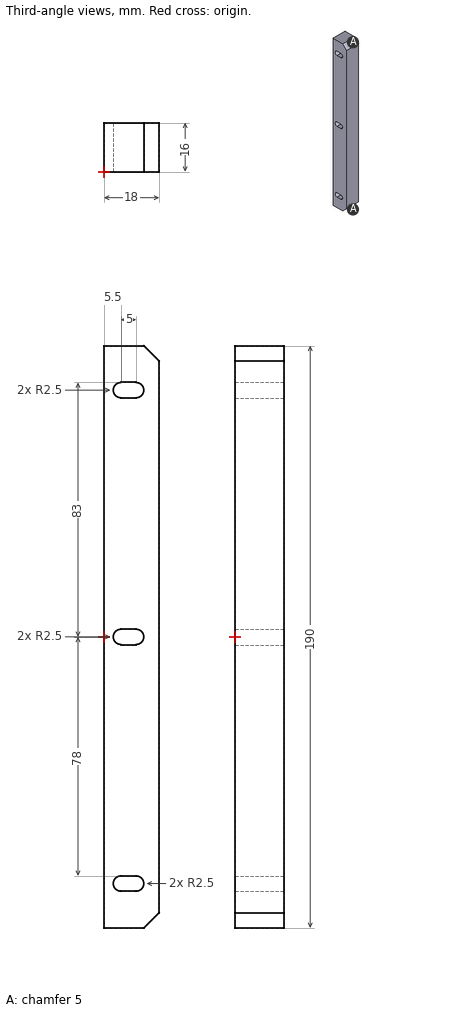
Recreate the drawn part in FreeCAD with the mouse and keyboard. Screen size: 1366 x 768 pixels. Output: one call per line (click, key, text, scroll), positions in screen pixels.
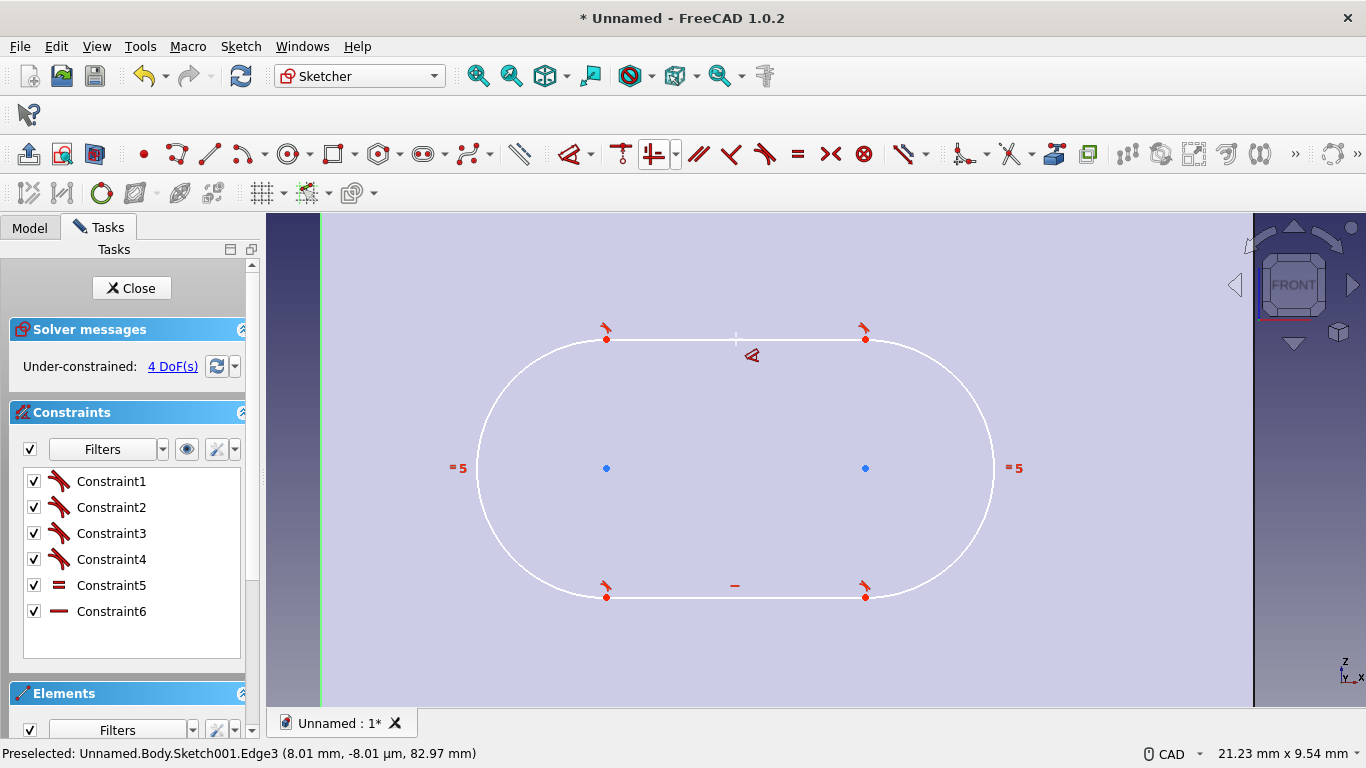
click(502, 393)
click(476, 374)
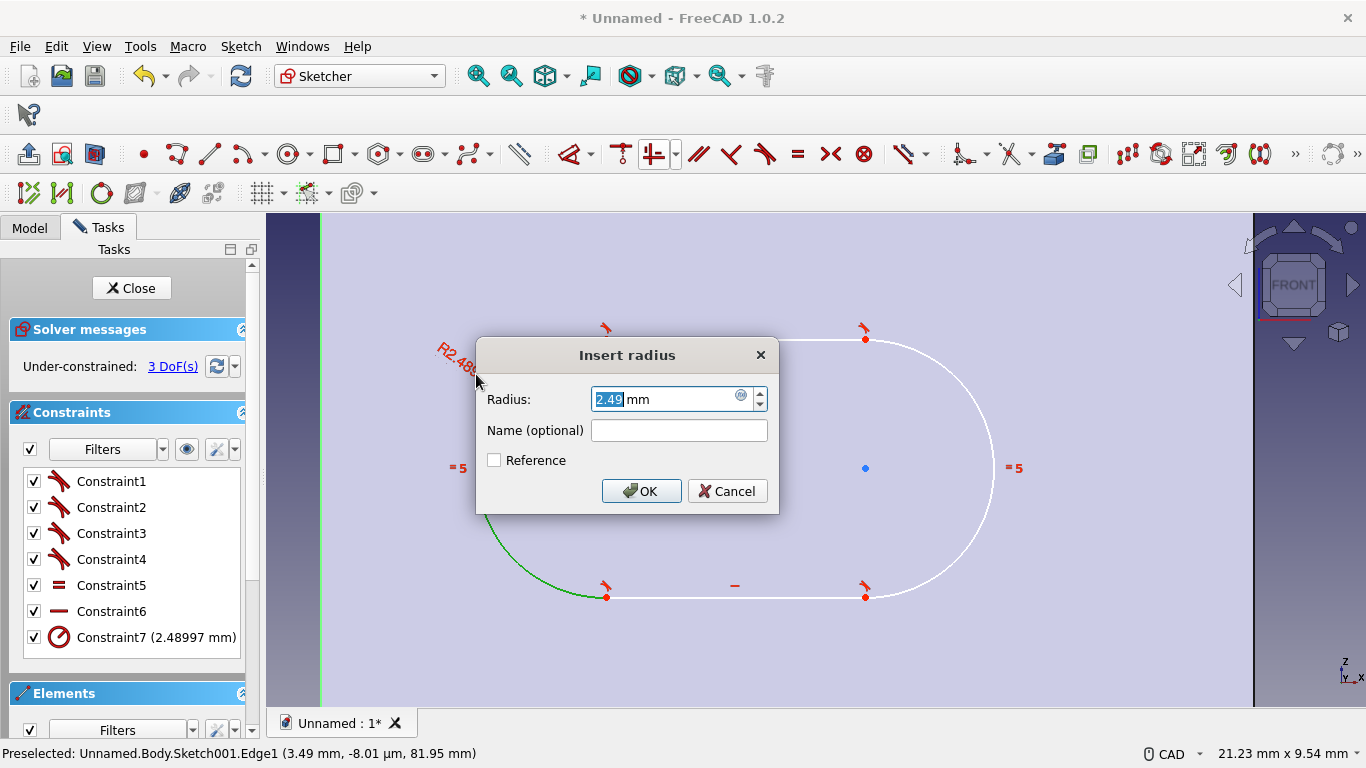
text(2.5)
key(Return)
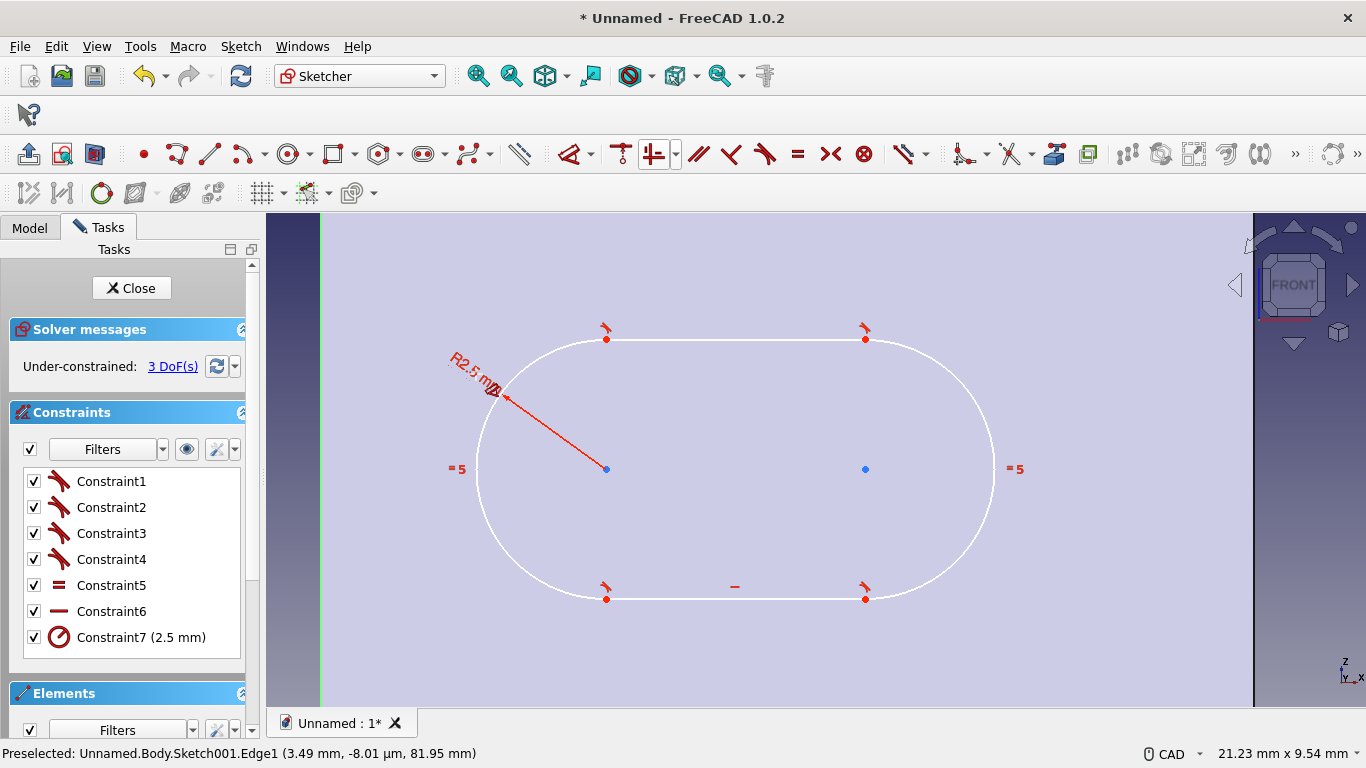
click(684, 340)
click(736, 306)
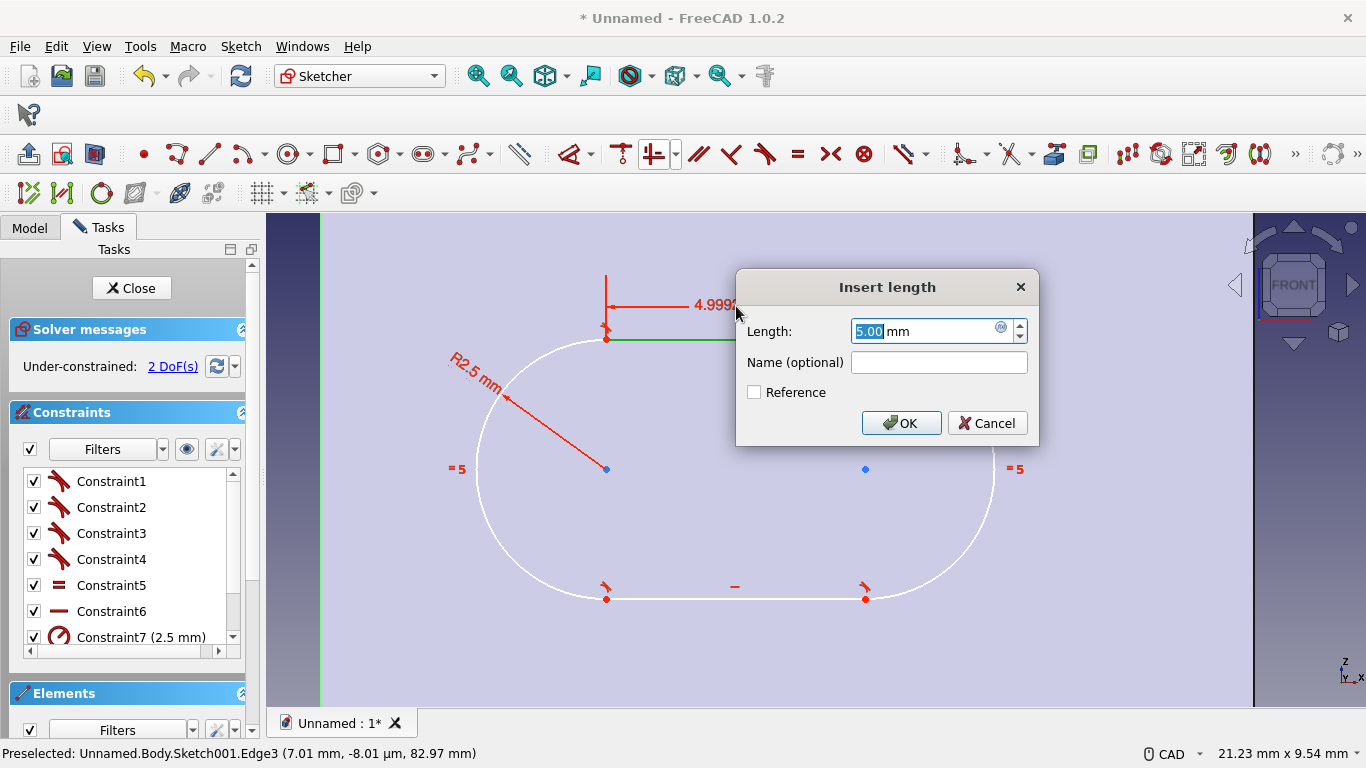
text(5)
key(Return)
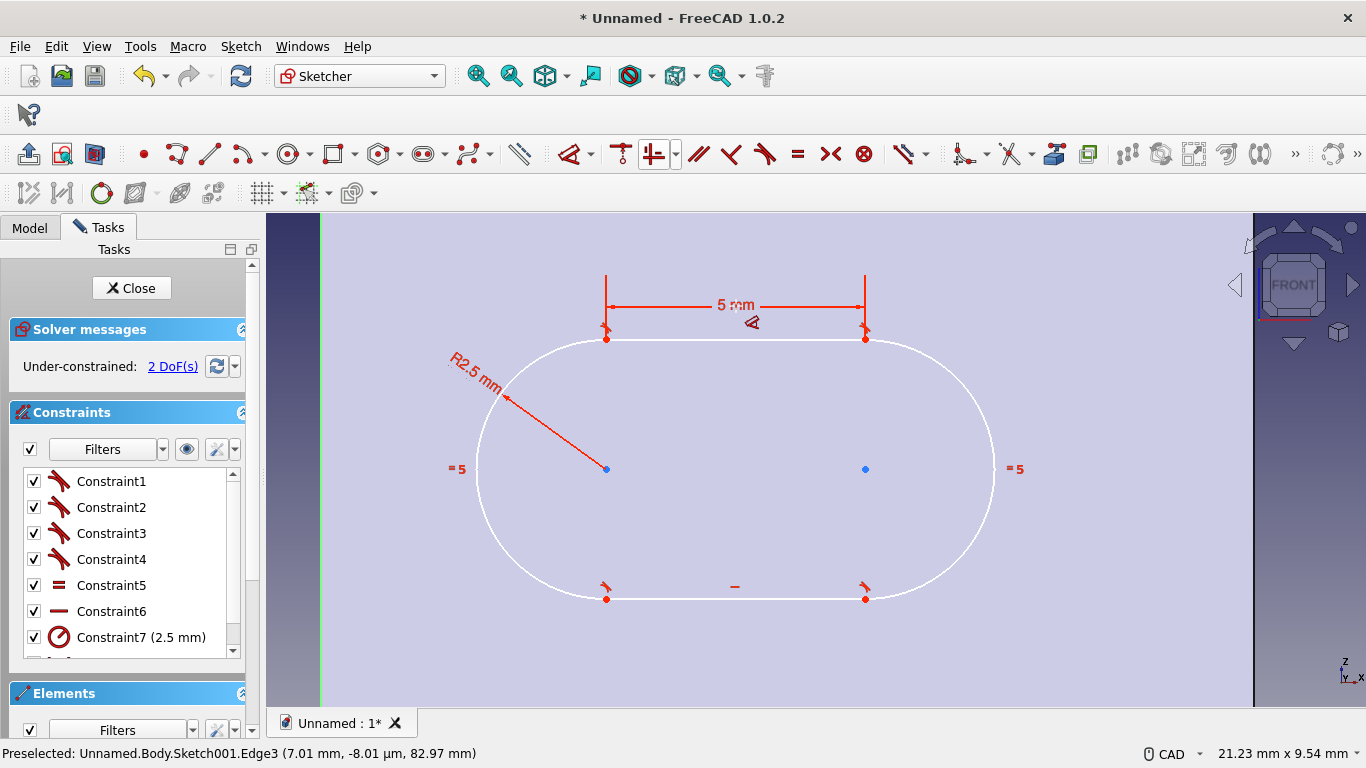
click(606, 340)
click(640, 509)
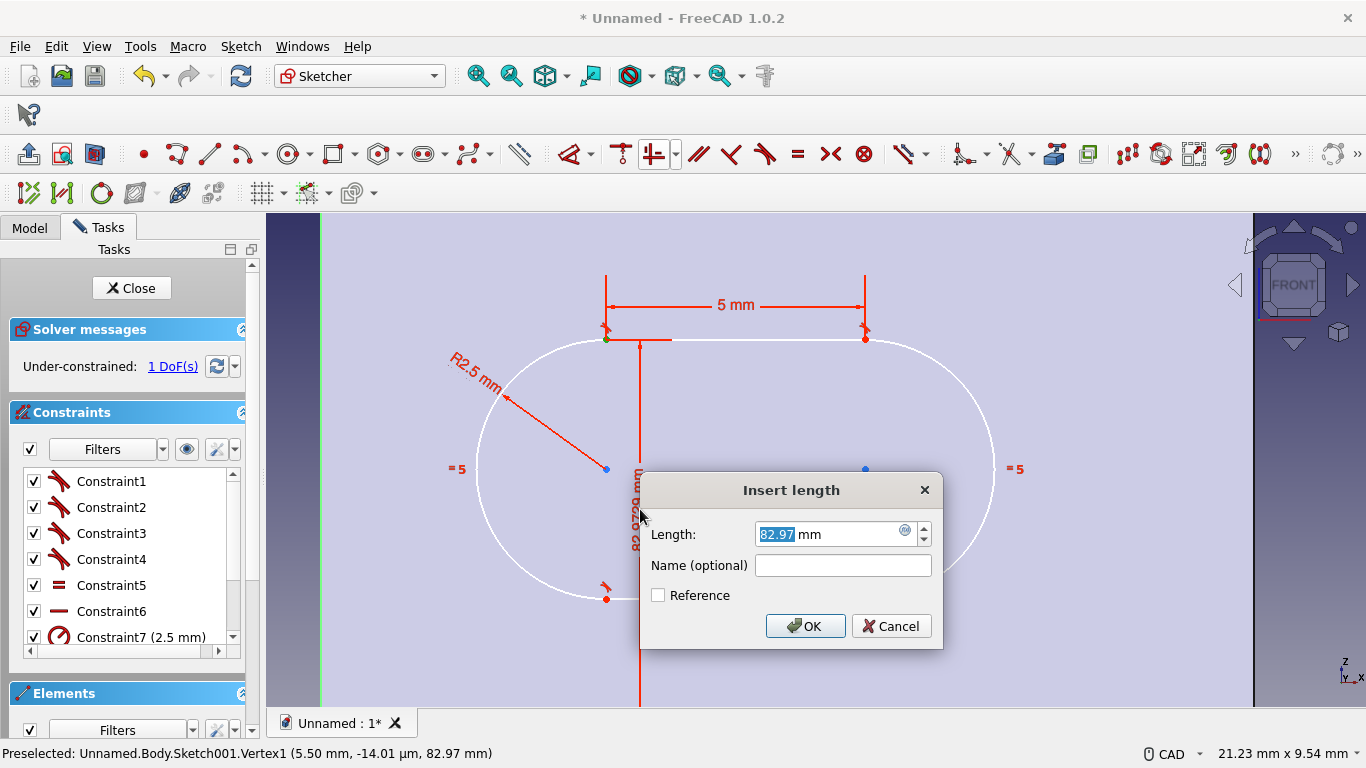
text(83)
key(Return)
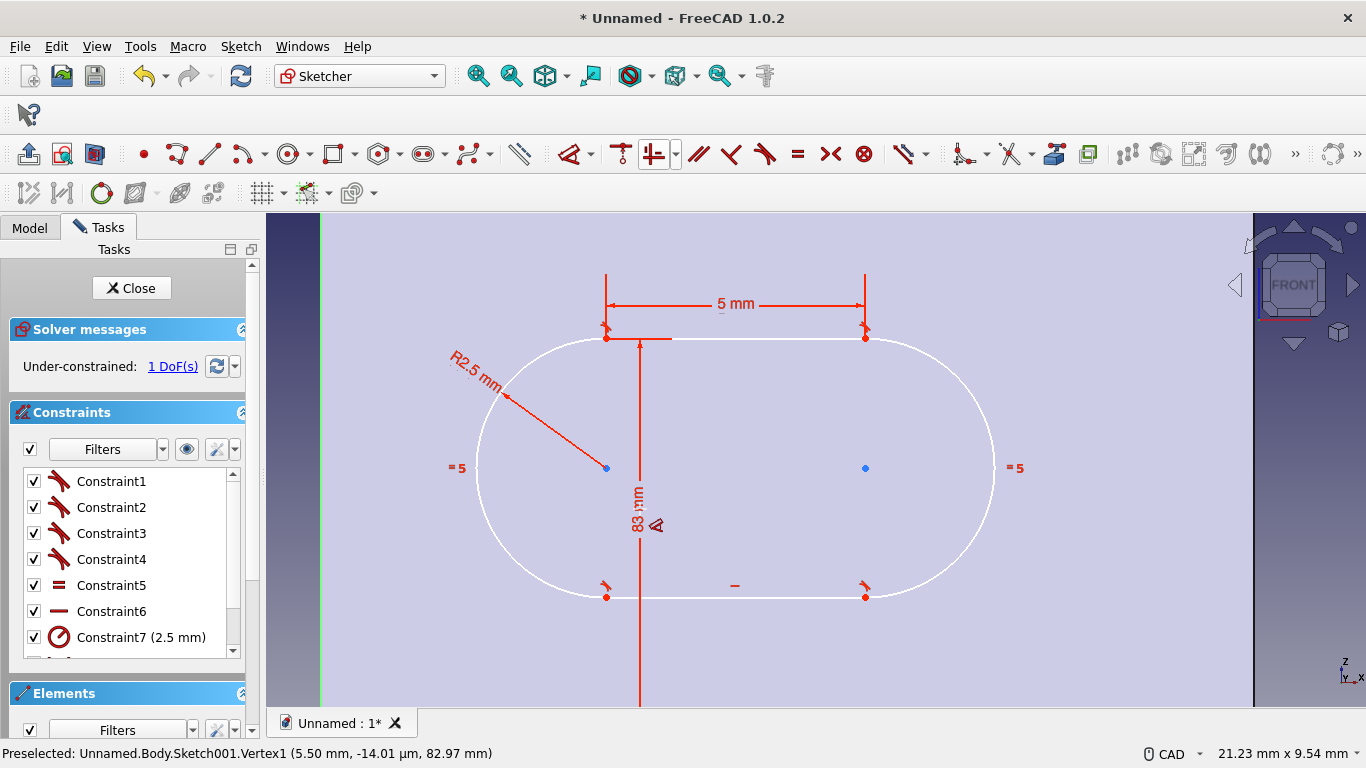
click(606, 339)
click(464, 305)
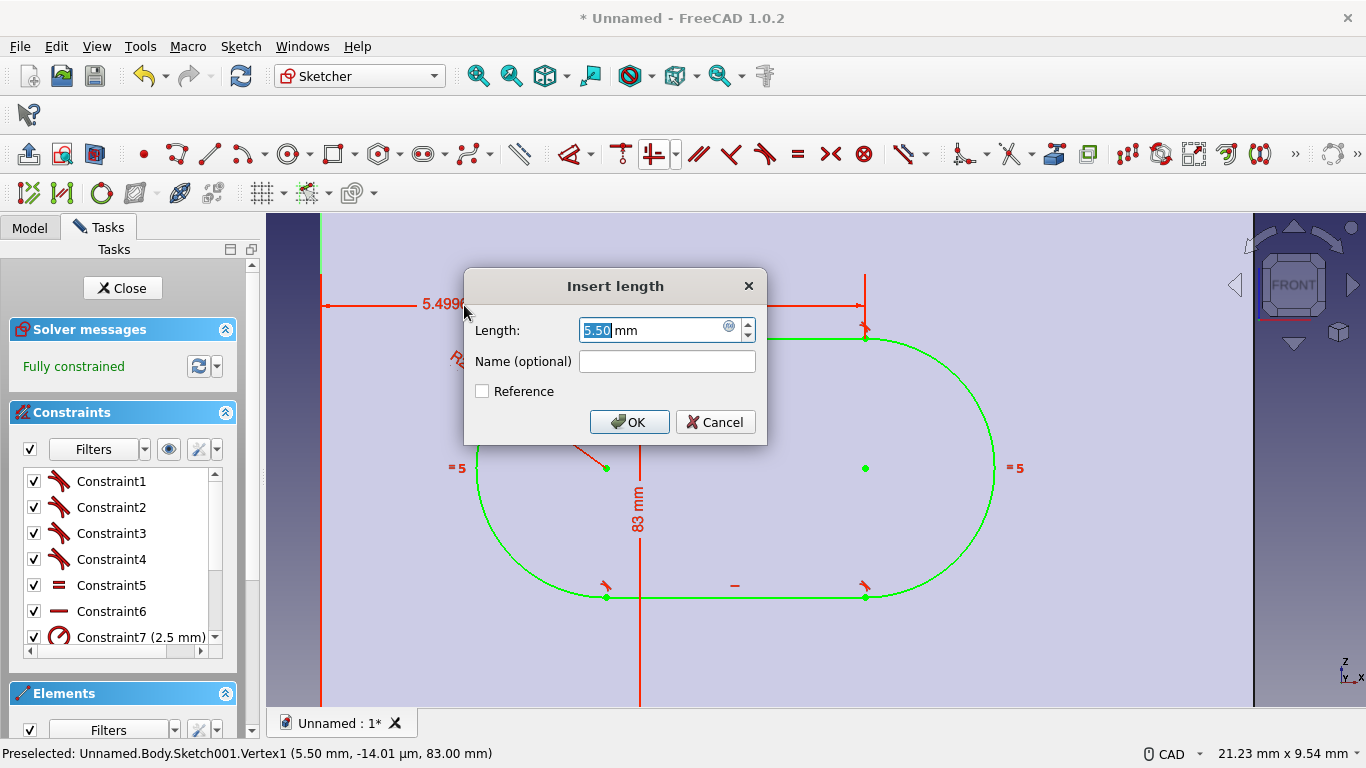
text(5.5)
key(Return)
key(Escape)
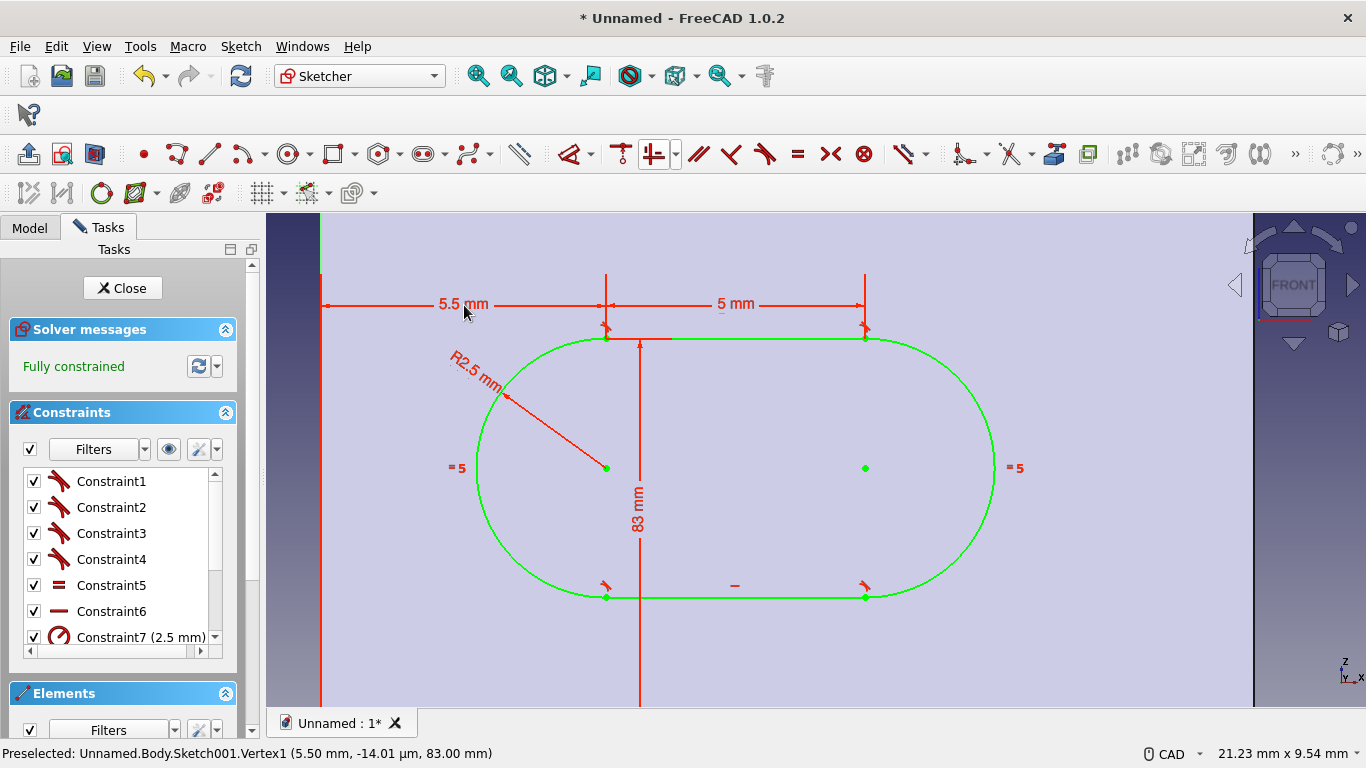
click(123, 288)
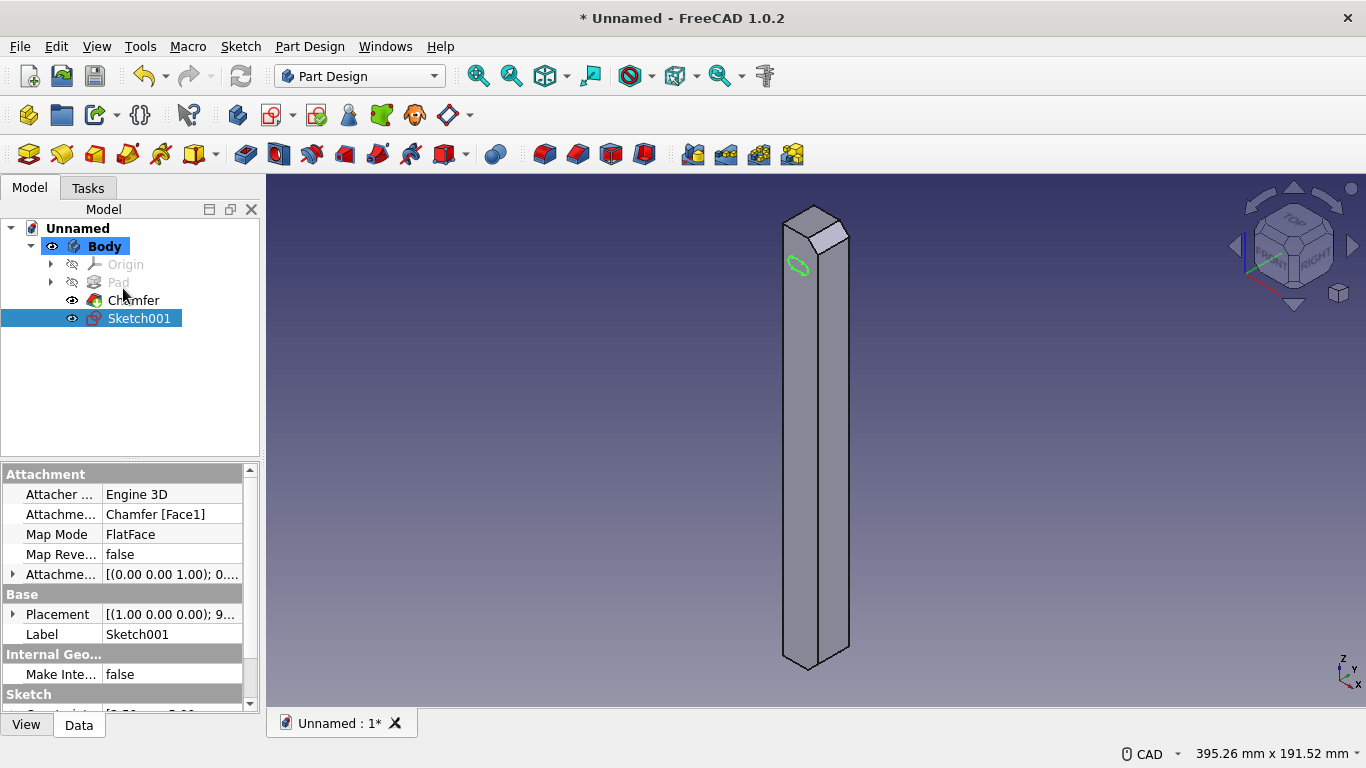
click(246, 154)